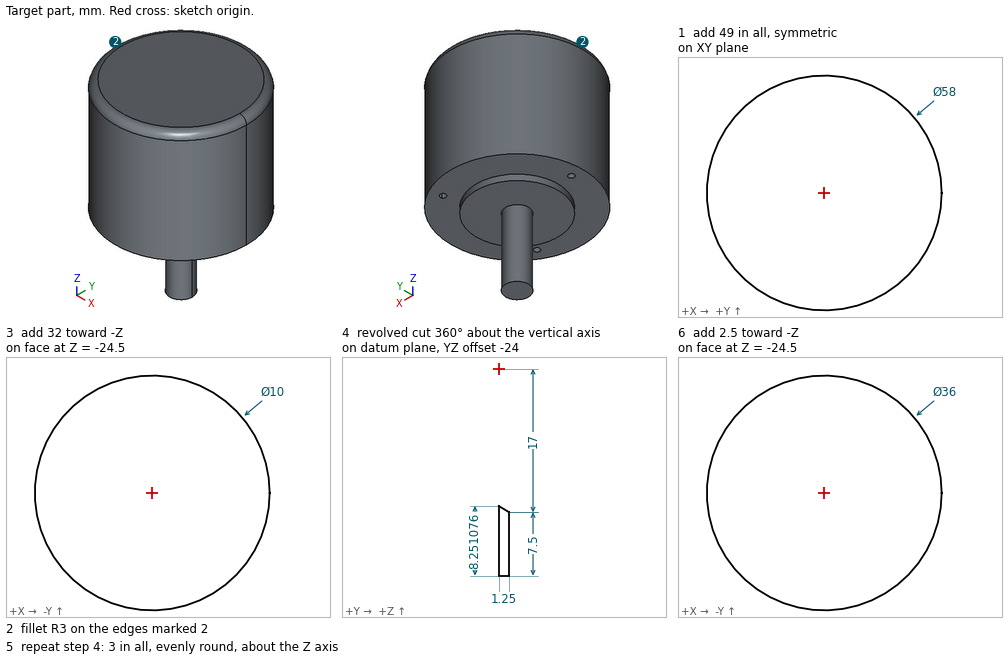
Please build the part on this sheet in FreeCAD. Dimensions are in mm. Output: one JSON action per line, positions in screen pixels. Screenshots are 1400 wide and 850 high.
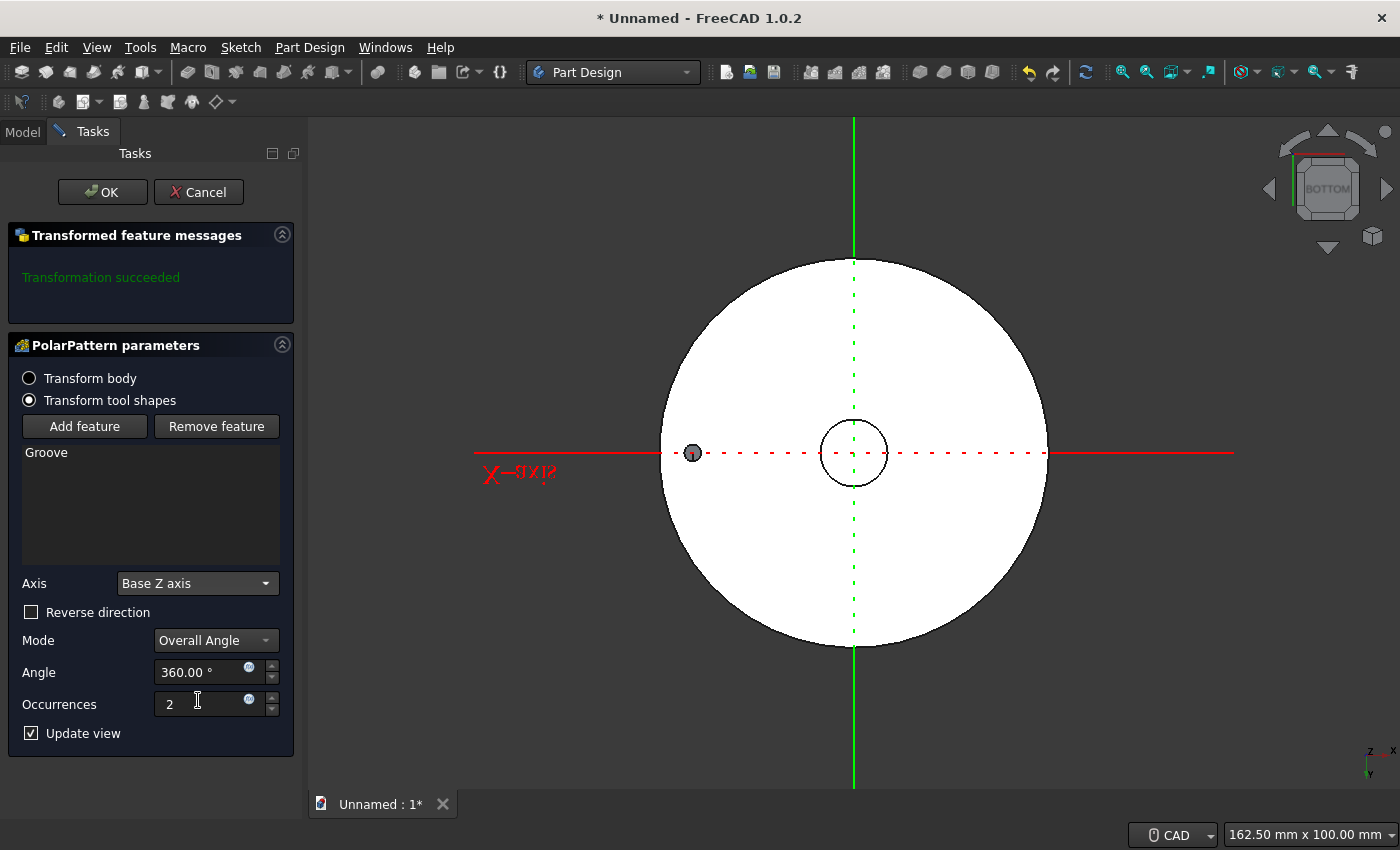
{"action": "triple_click", "coordinate": [209, 704]}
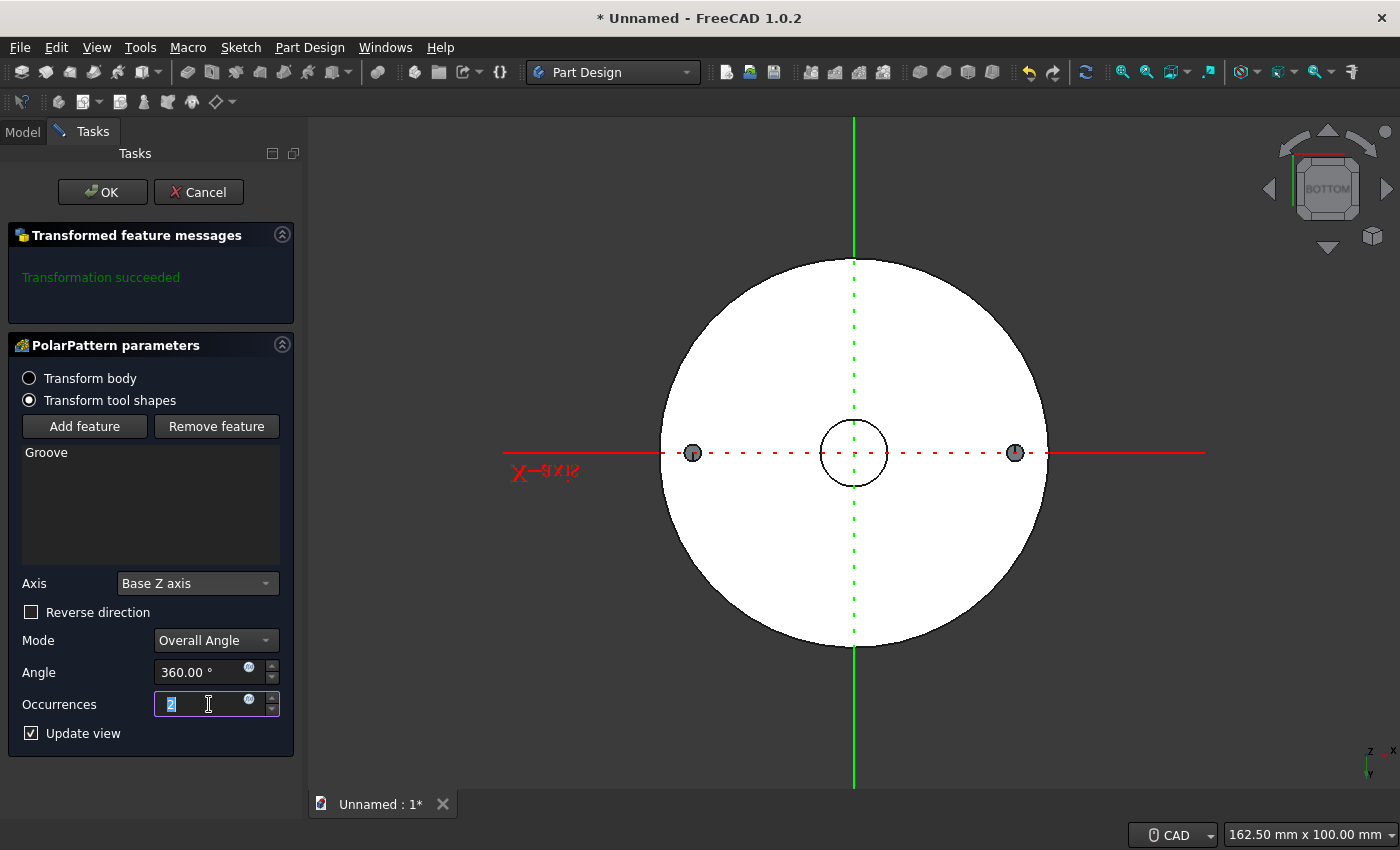
{"action": "type", "text": "3"}
{"action": "key", "text": "Tab"}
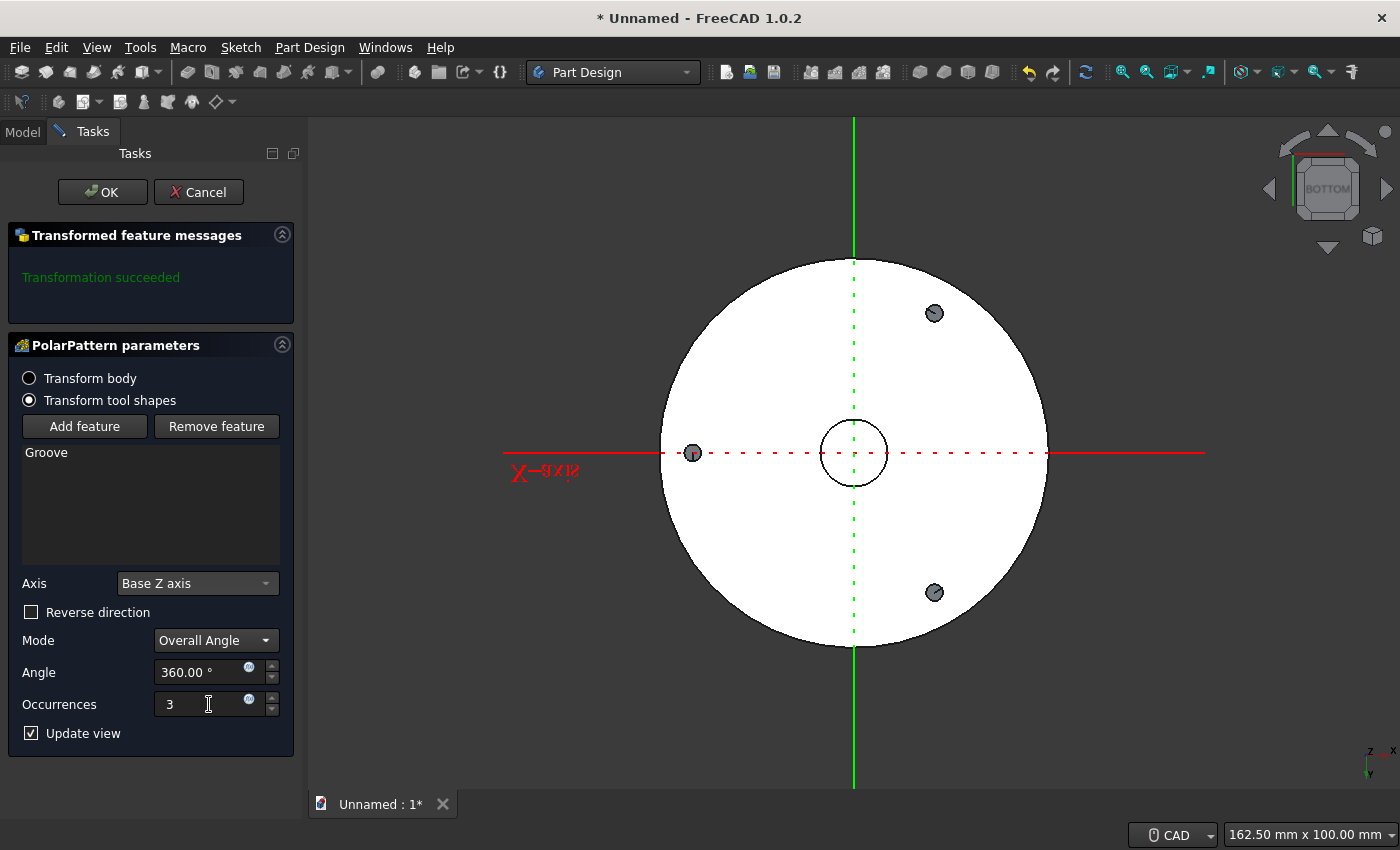
{"action": "left_click", "coordinate": [103, 192]}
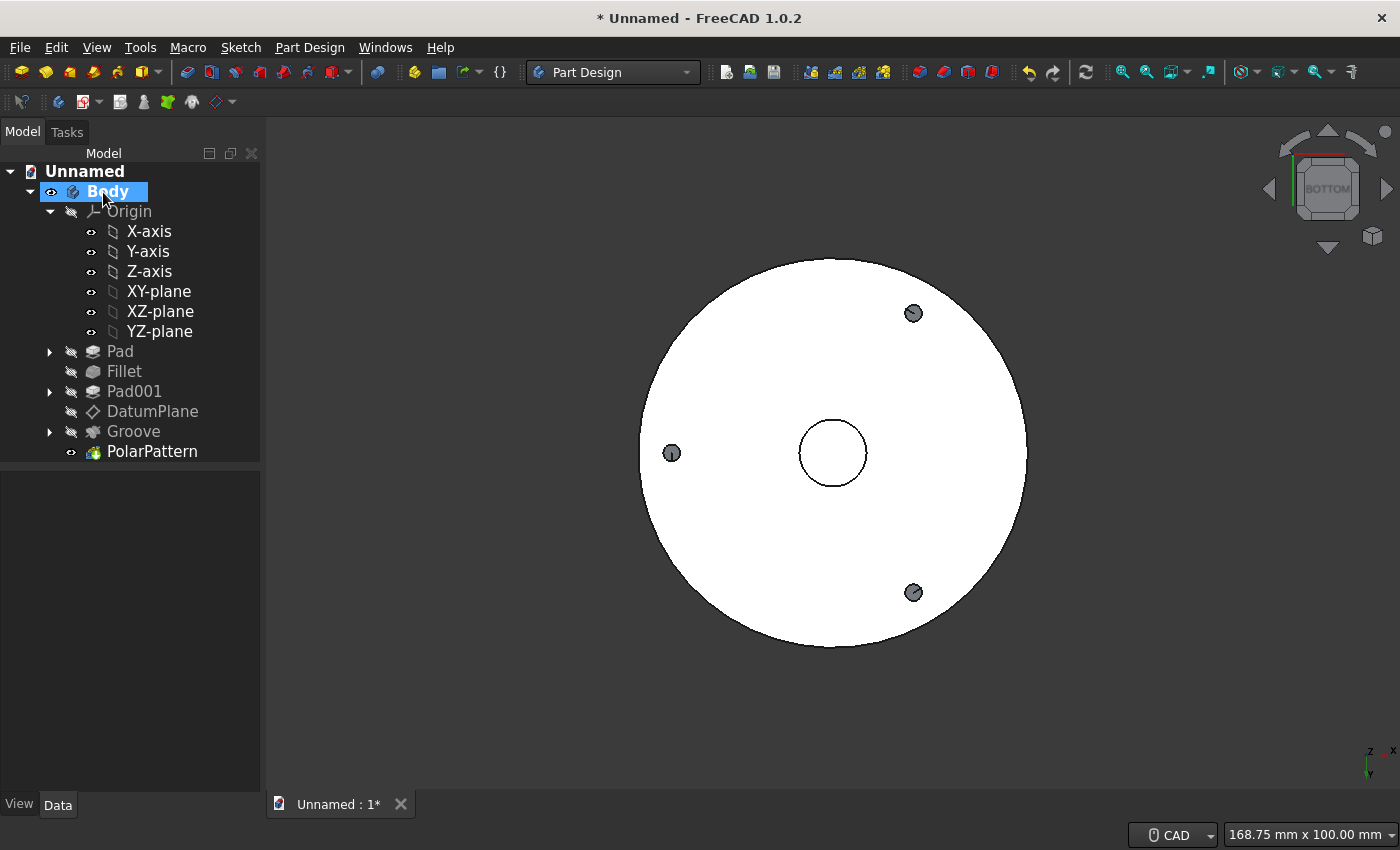
{"action": "left_click", "coordinate": [944, 452]}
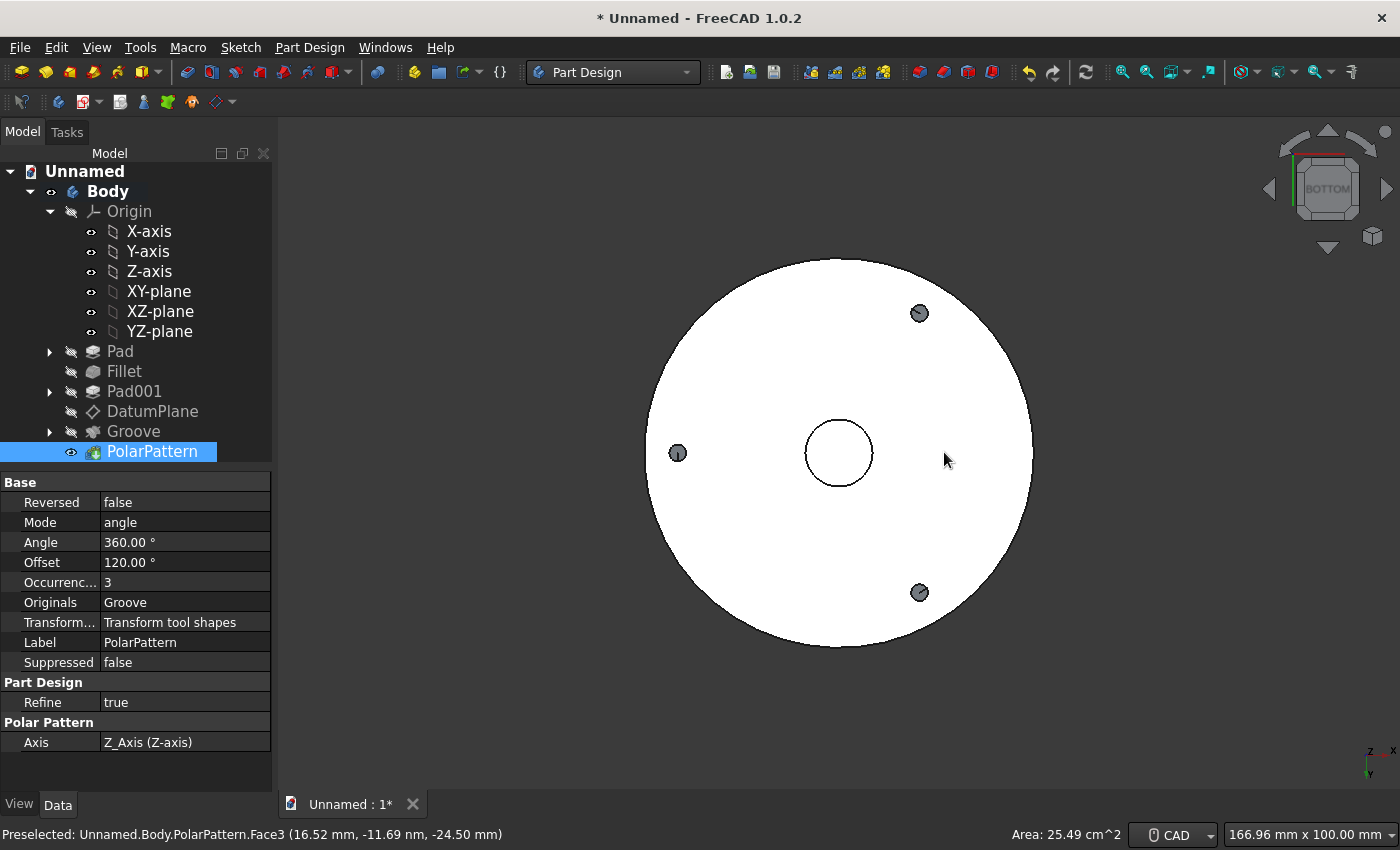
{"action": "left_click", "coordinate": [84, 102]}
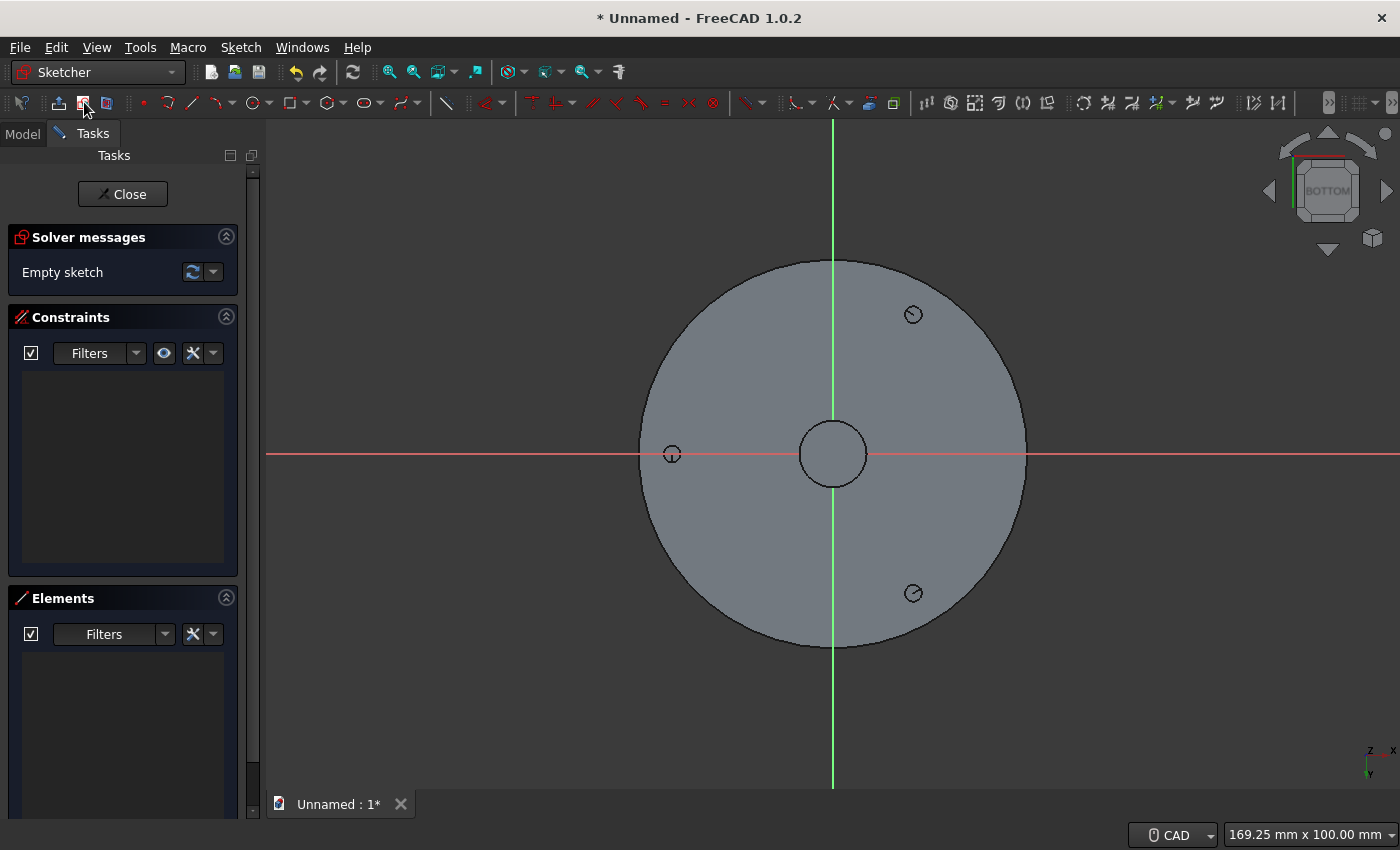
{"action": "scroll", "coordinate": [916, 454], "scroll_direction": "up", "scroll_amount": 3}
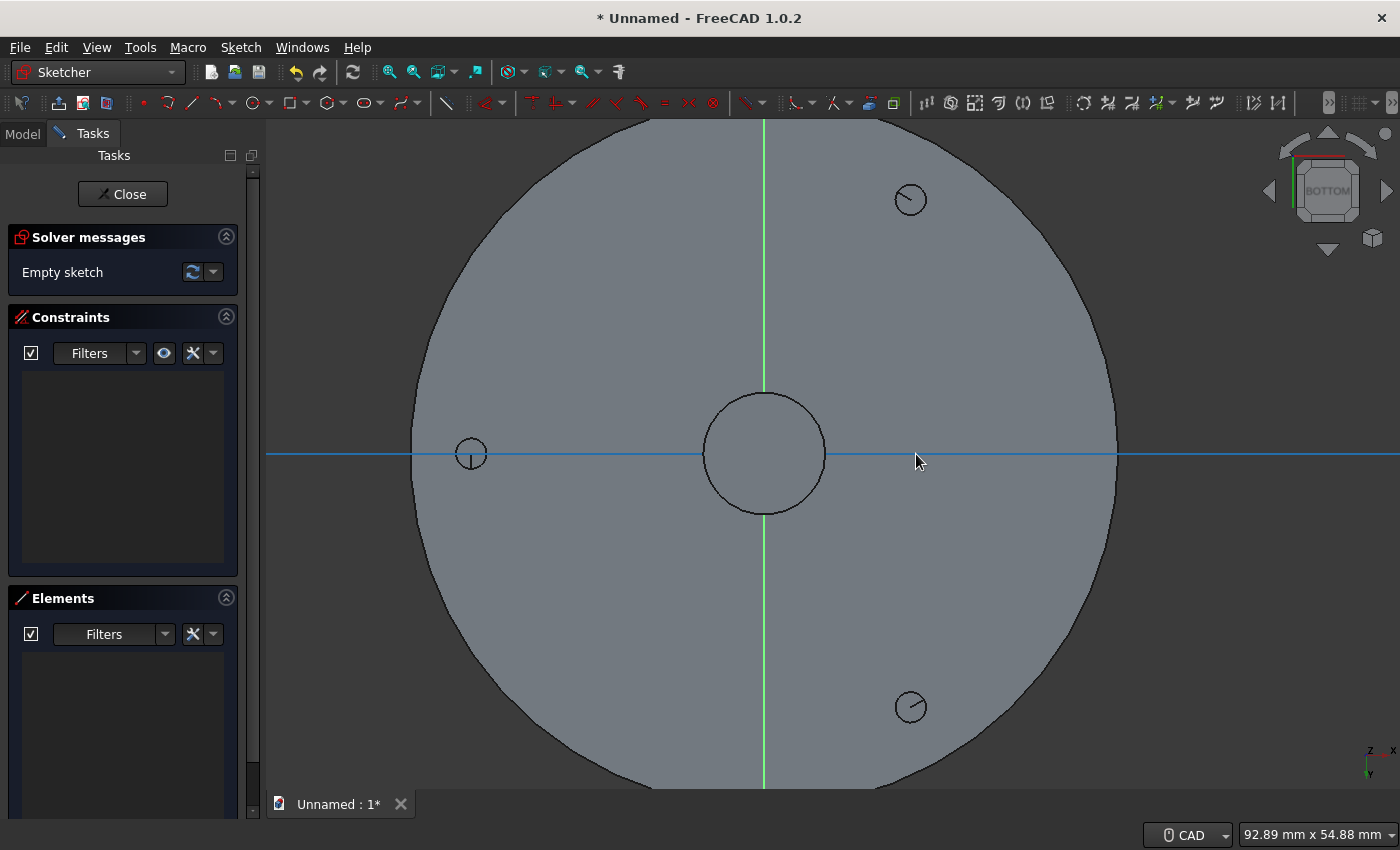
{"action": "left_click", "coordinate": [254, 104]}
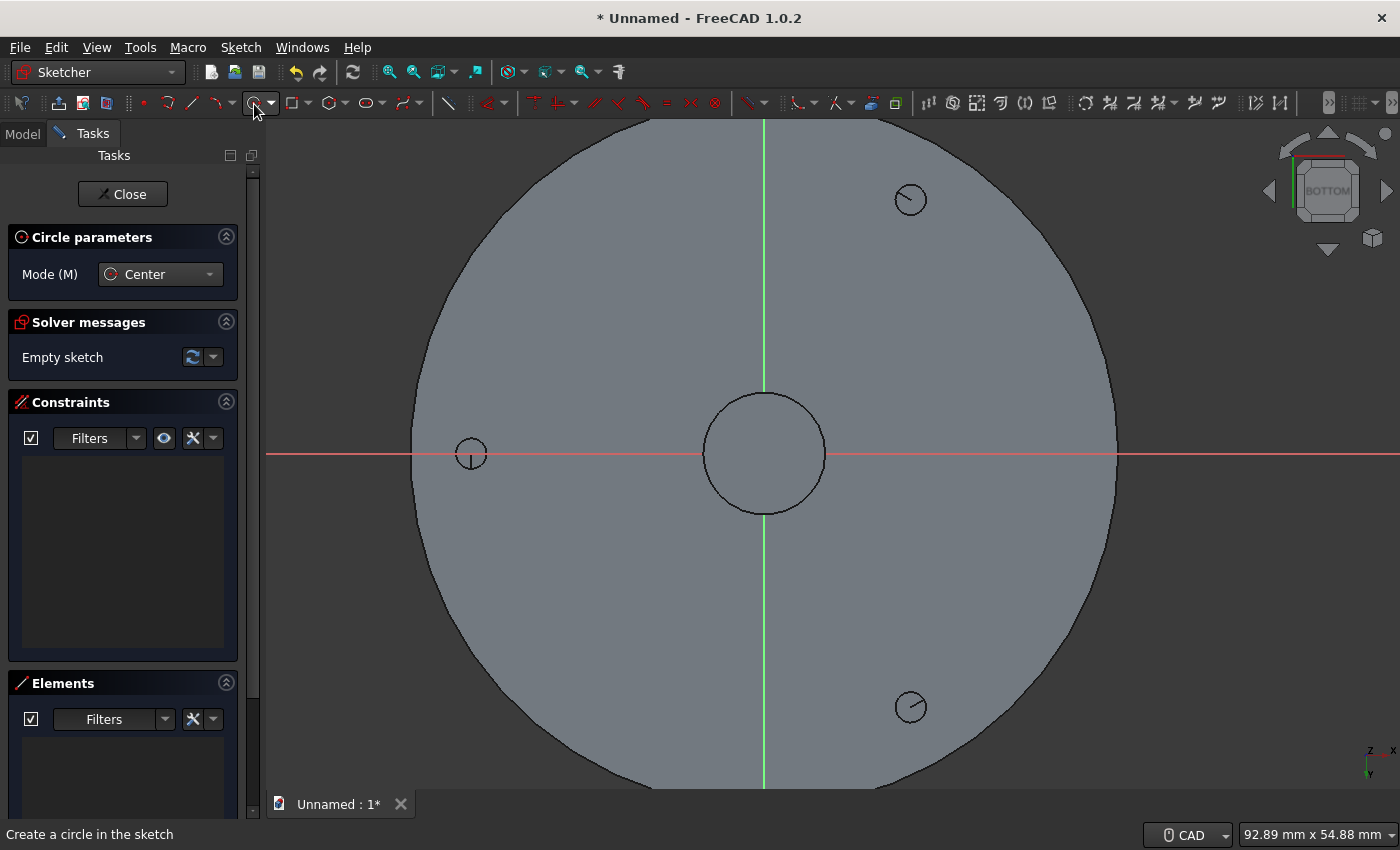
{"action": "left_click", "coordinate": [764, 454]}
{"action": "left_click", "coordinate": [920, 298]}
{"action": "key", "text": "Escape"}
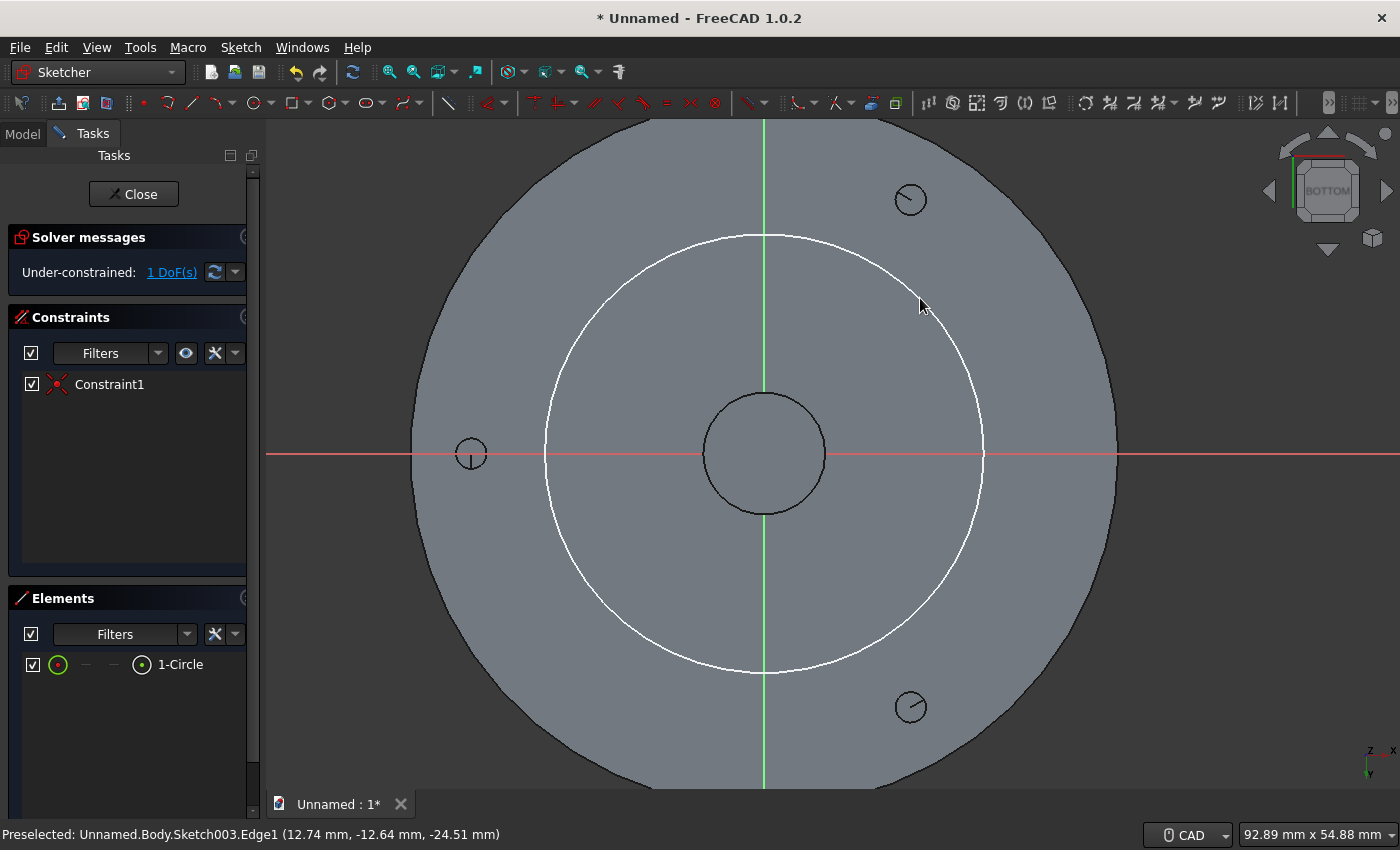
{"action": "left_click", "coordinate": [488, 104]}